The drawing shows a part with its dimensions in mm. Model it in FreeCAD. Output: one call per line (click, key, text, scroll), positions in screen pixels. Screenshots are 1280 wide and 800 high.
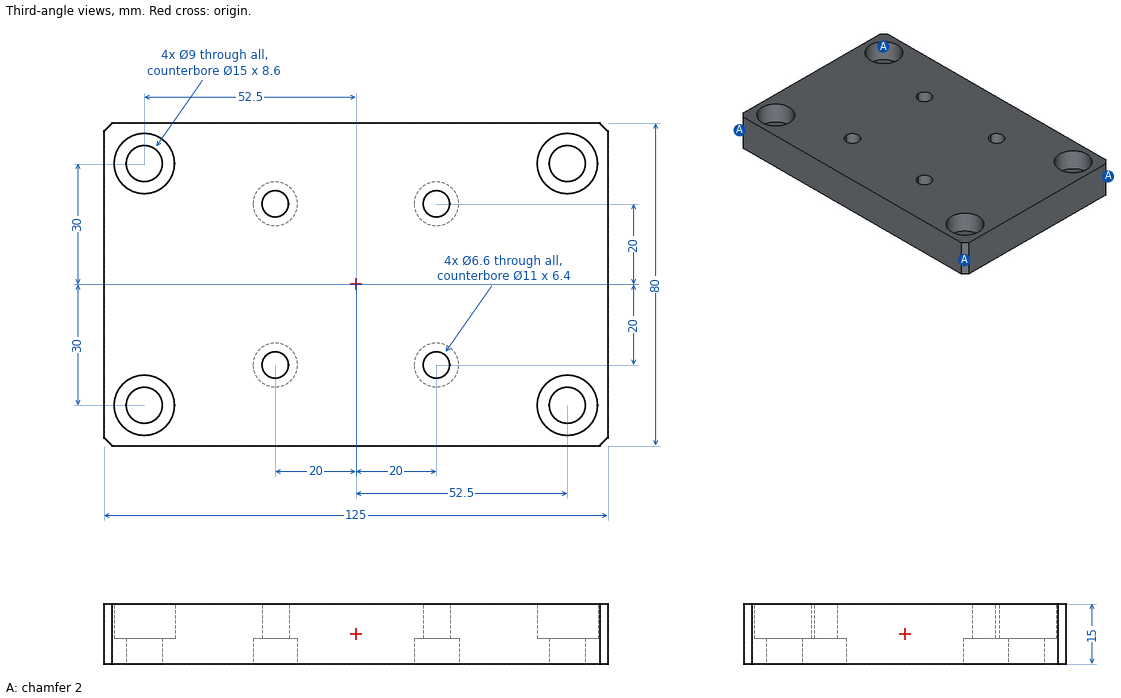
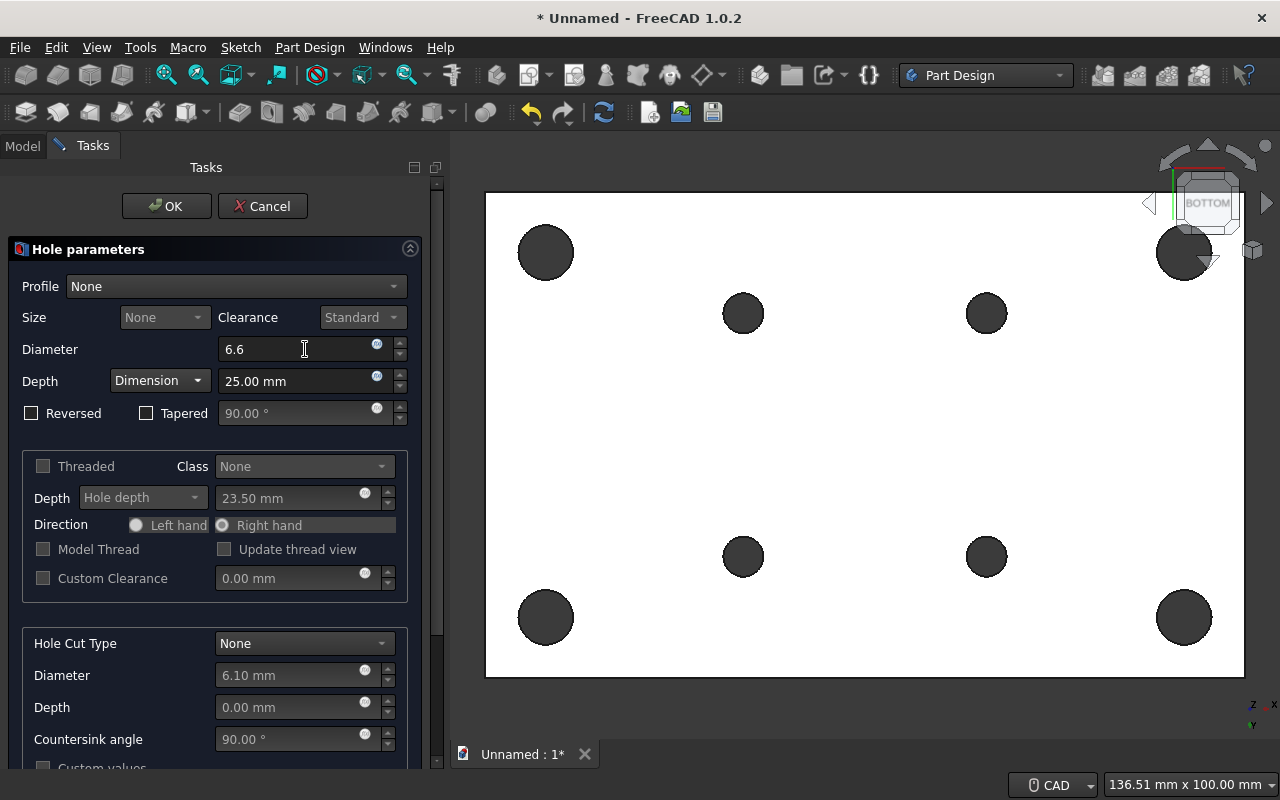
click(161, 380)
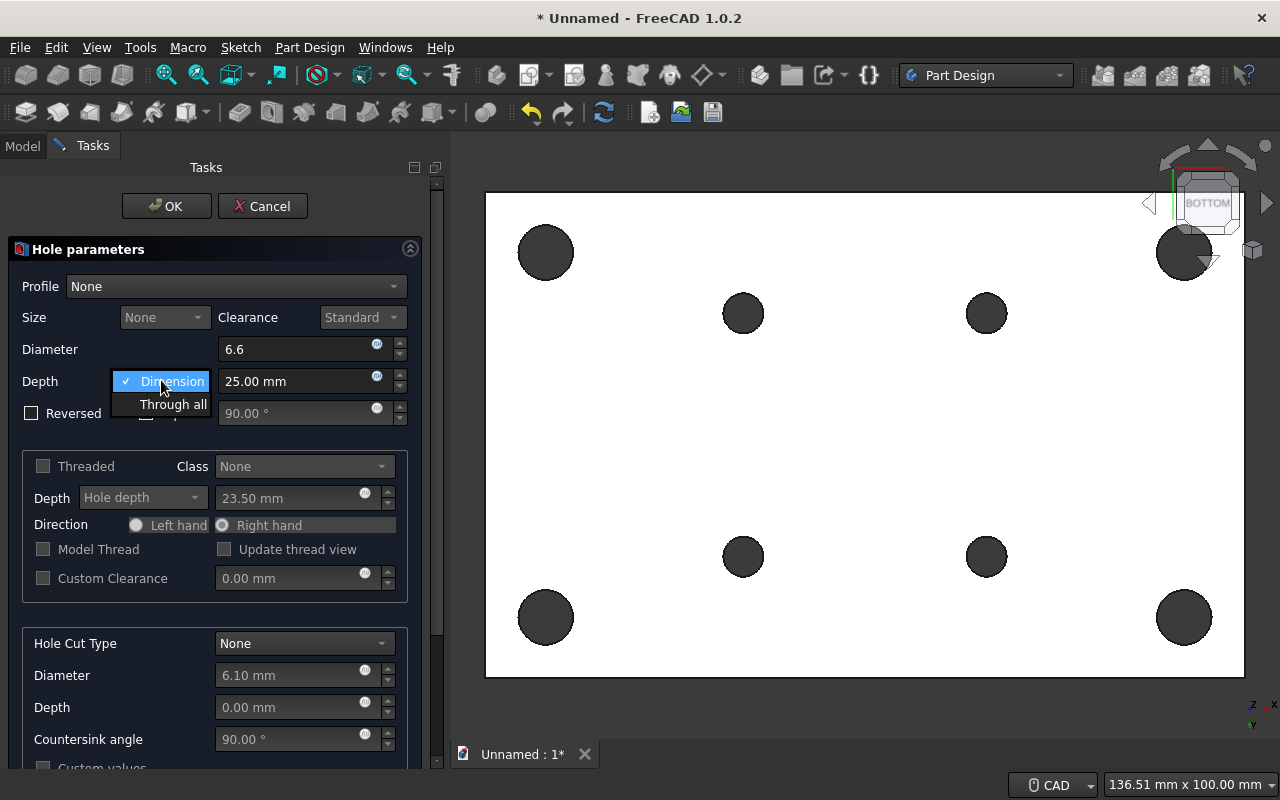
click(160, 404)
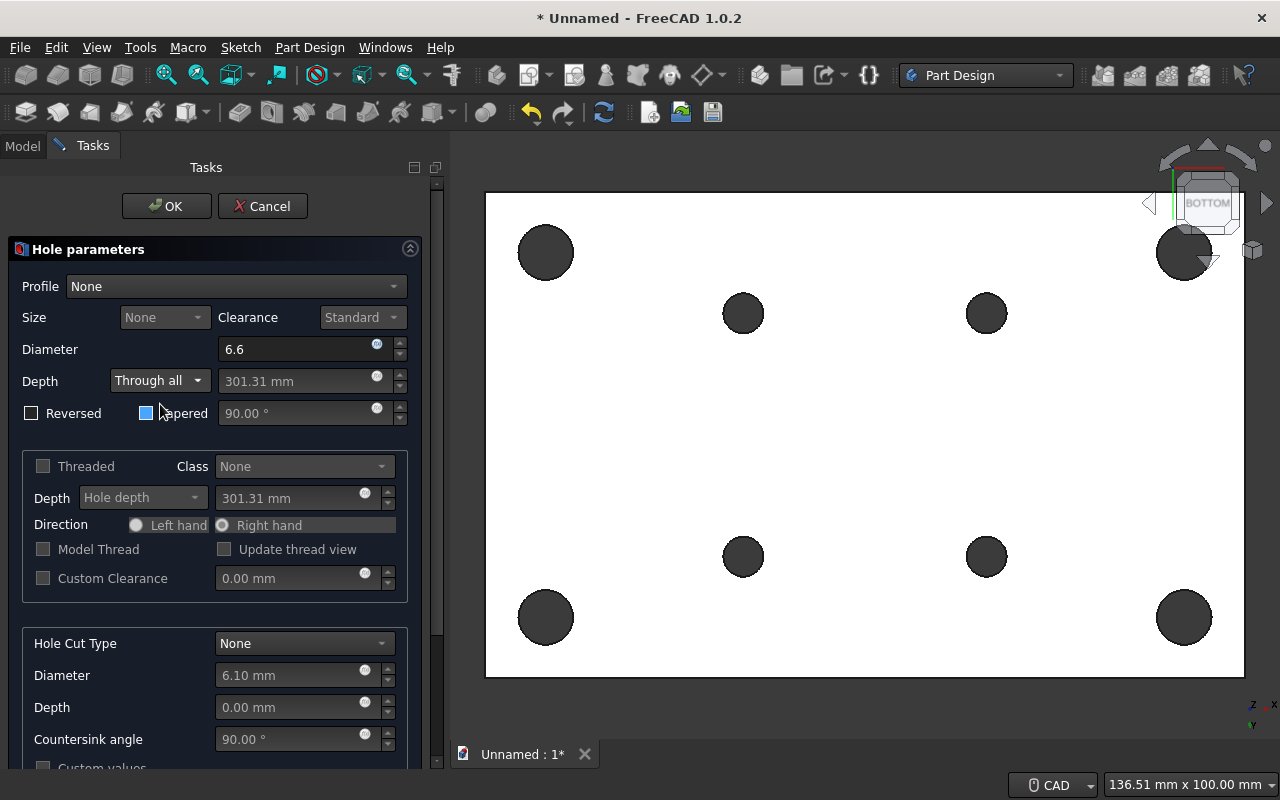
click(306, 644)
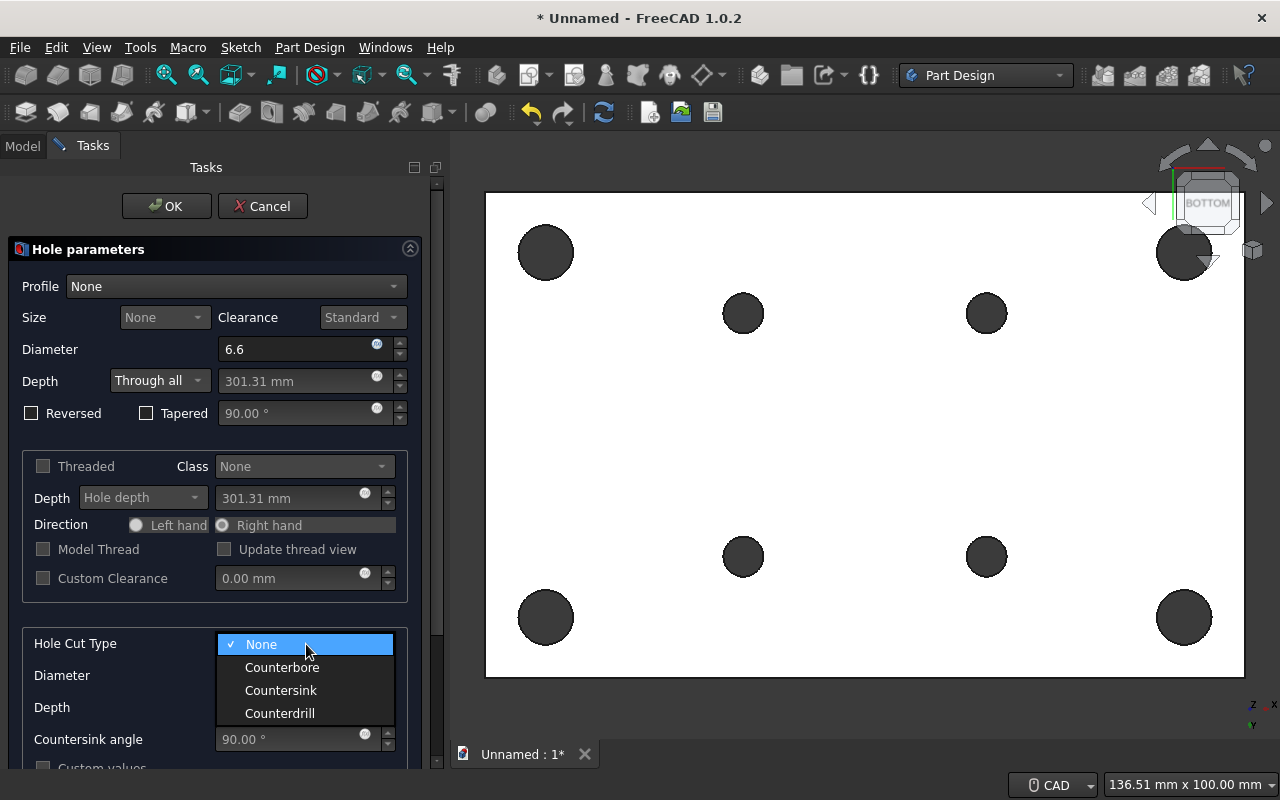
click(304, 668)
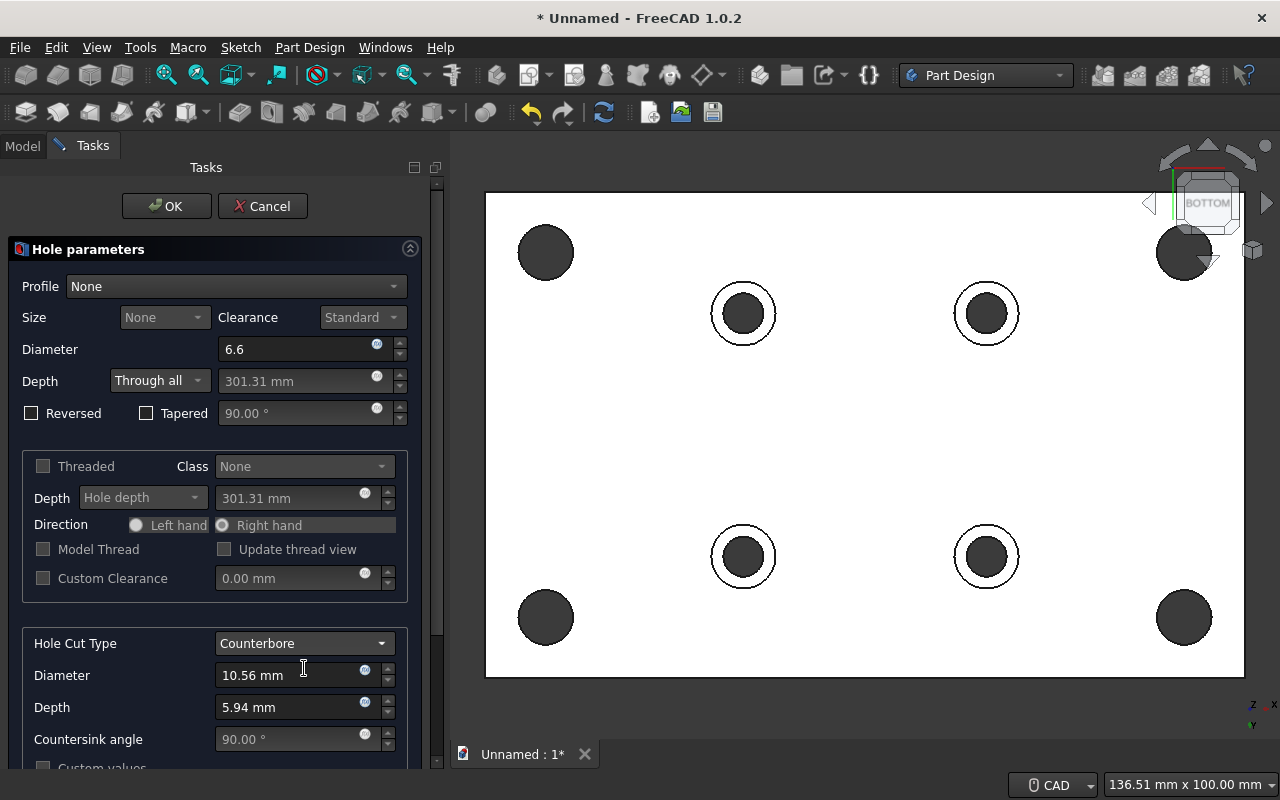
triple_click(298, 675)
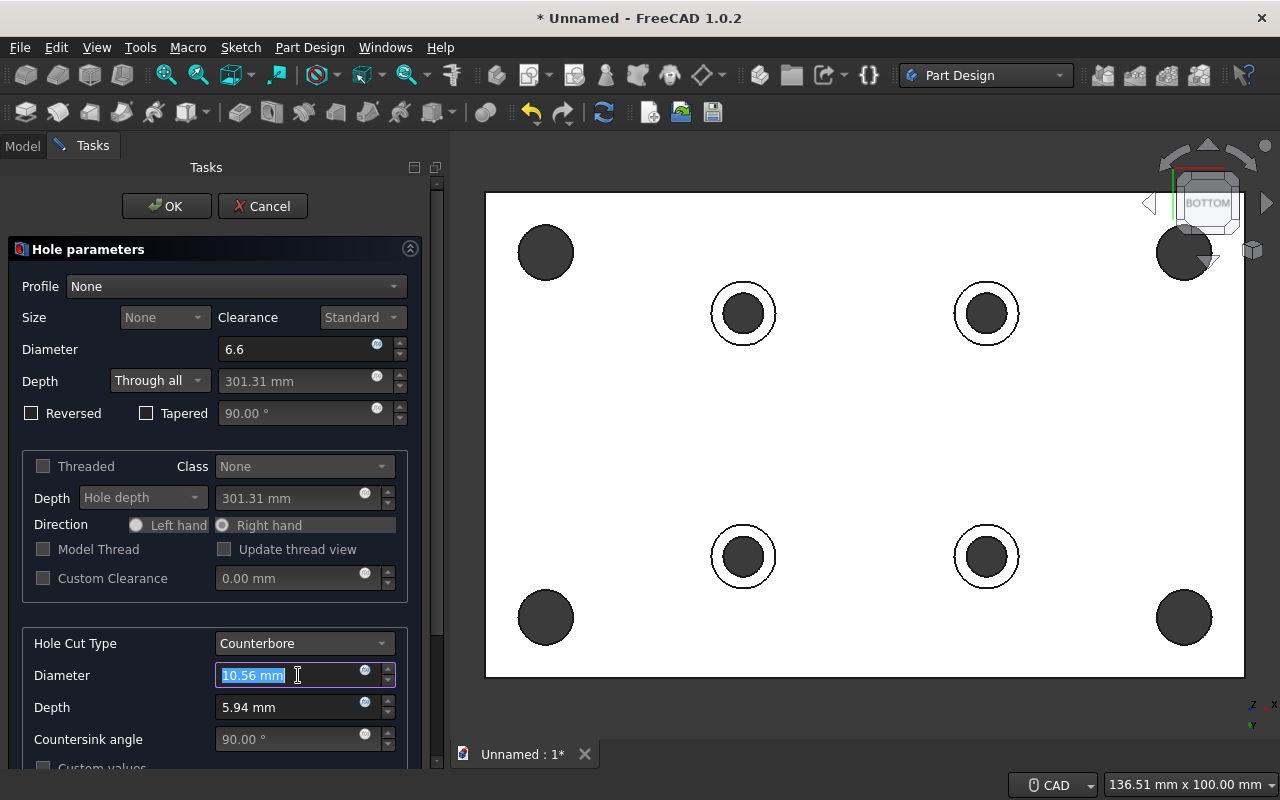
text(11)
key(Tab)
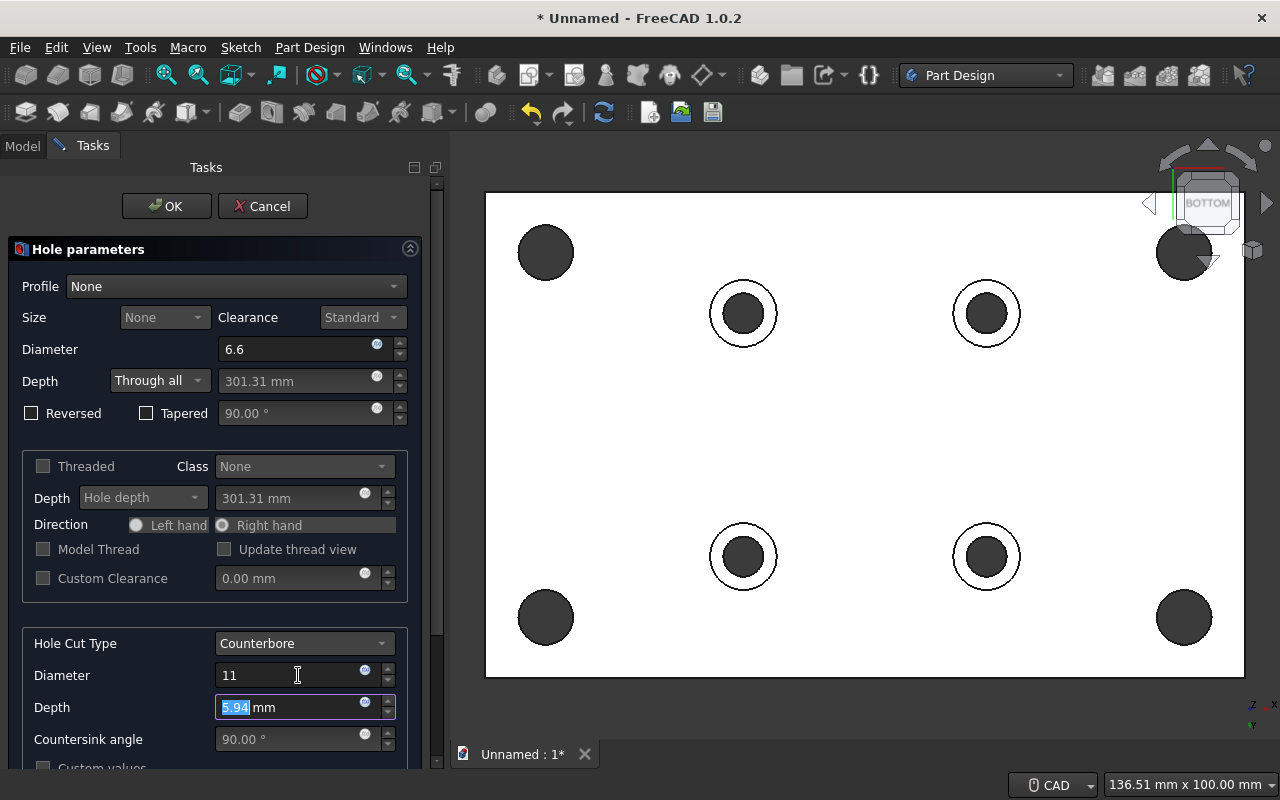
text(6.4)
key(Tab)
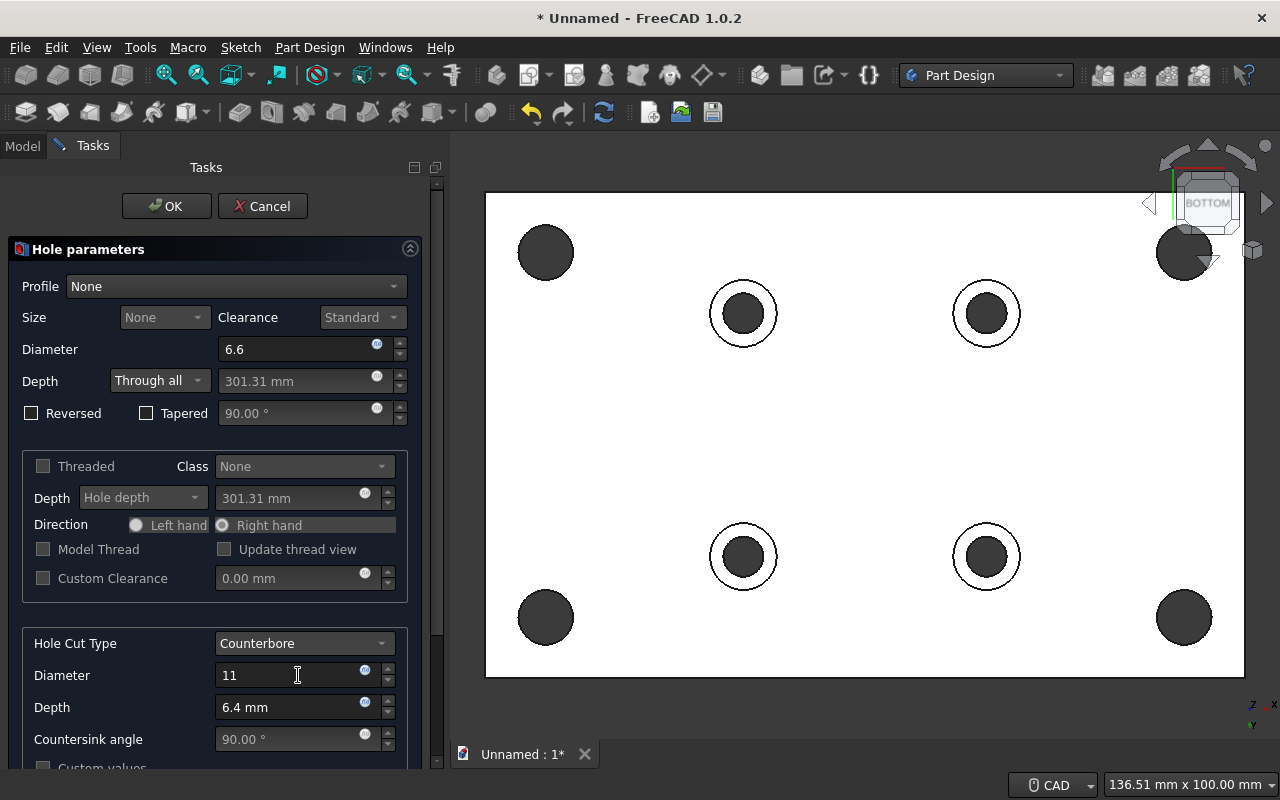
click(167, 206)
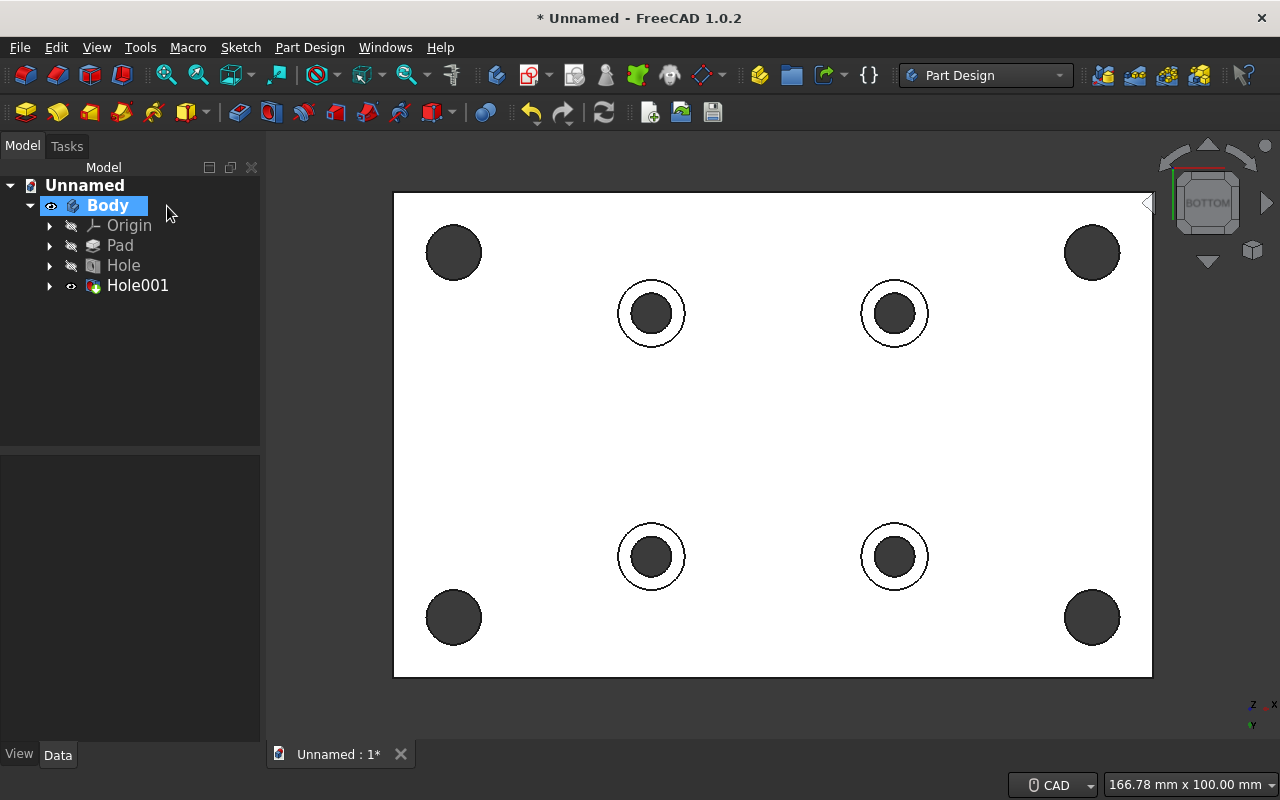
key(0)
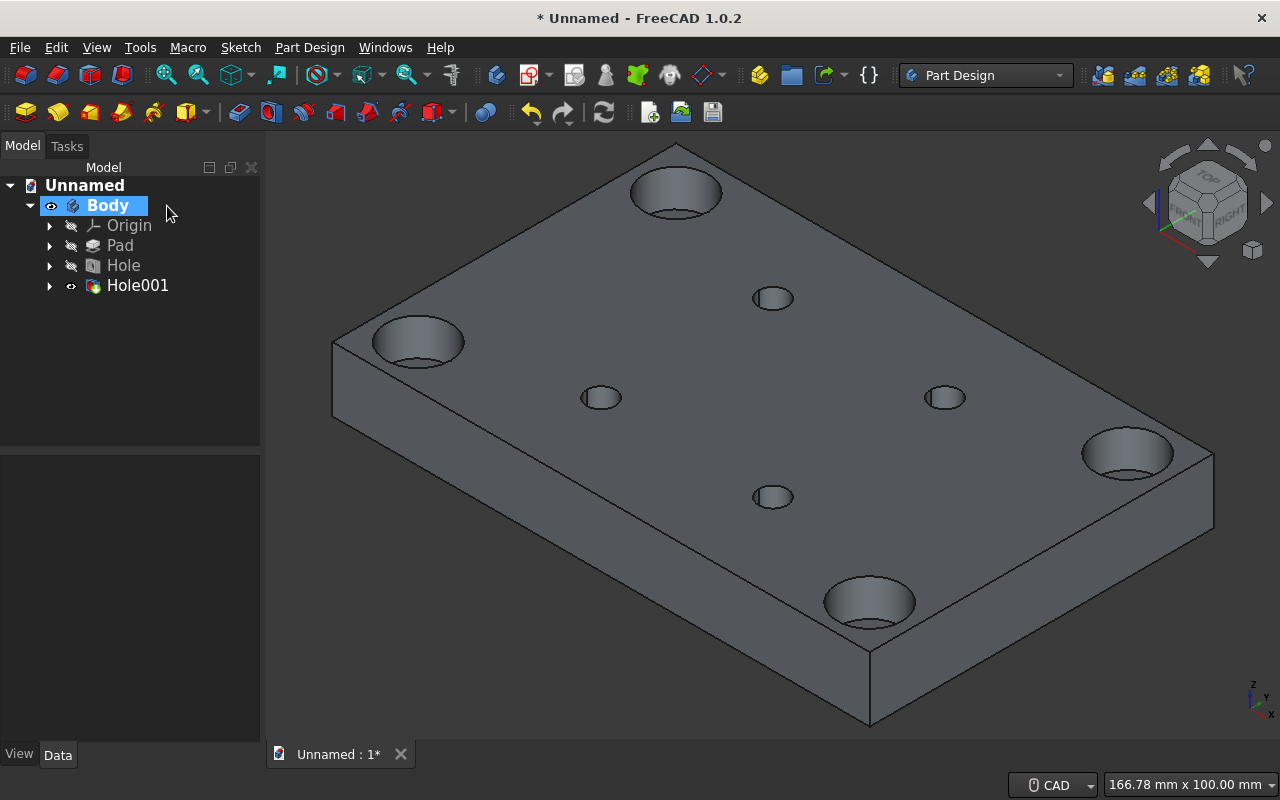
click(870, 688)